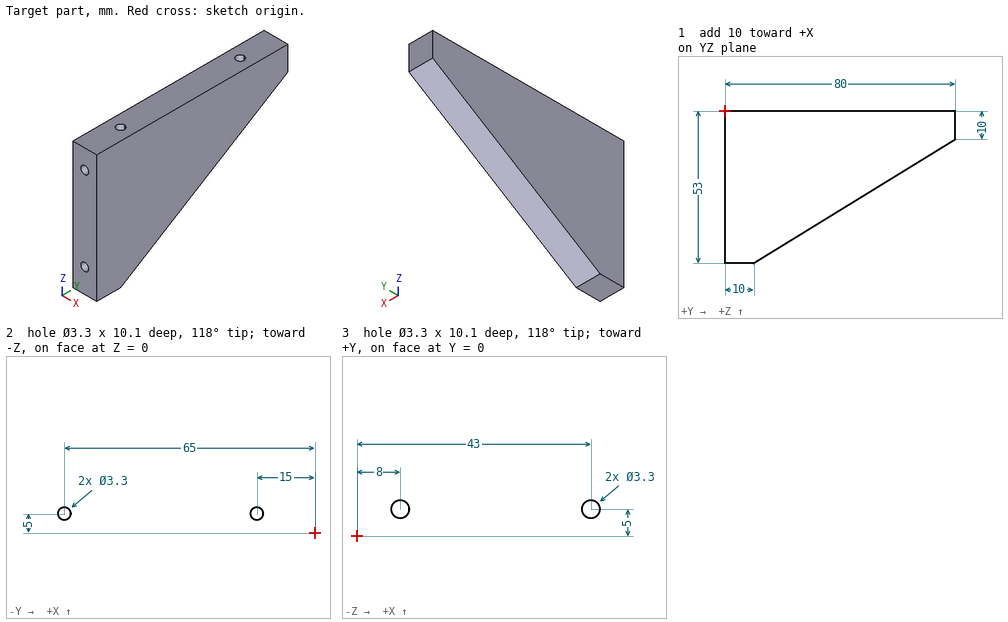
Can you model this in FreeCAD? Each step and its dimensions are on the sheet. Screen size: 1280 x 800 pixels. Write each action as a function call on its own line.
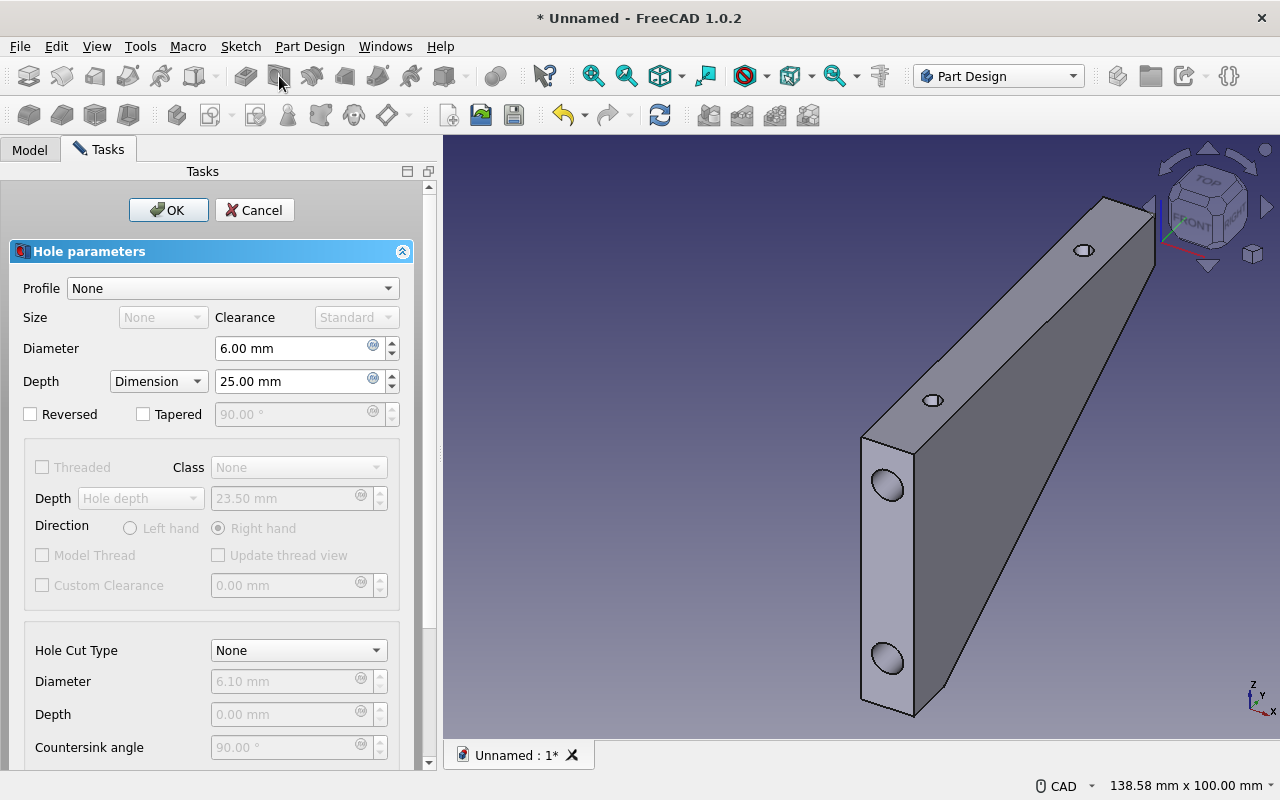
triple_click(300, 348)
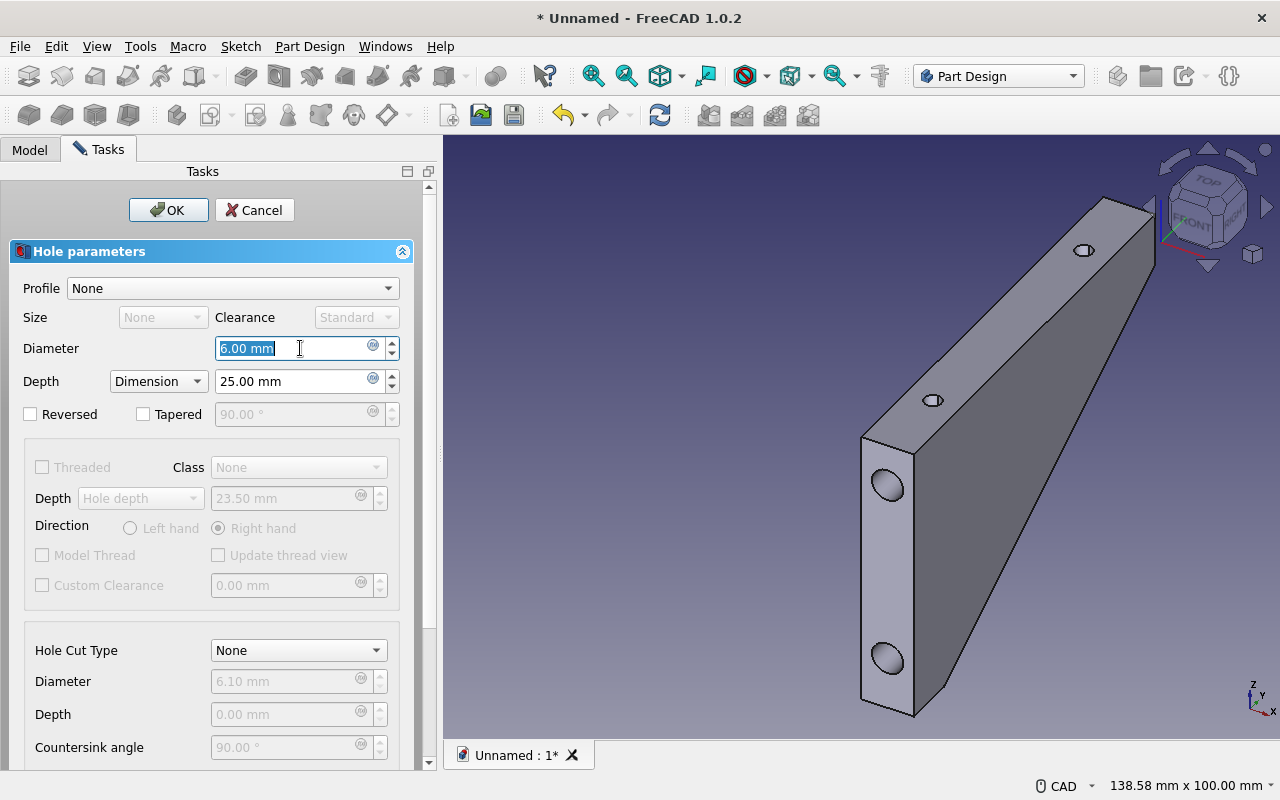
text(3.3)
key(Tab)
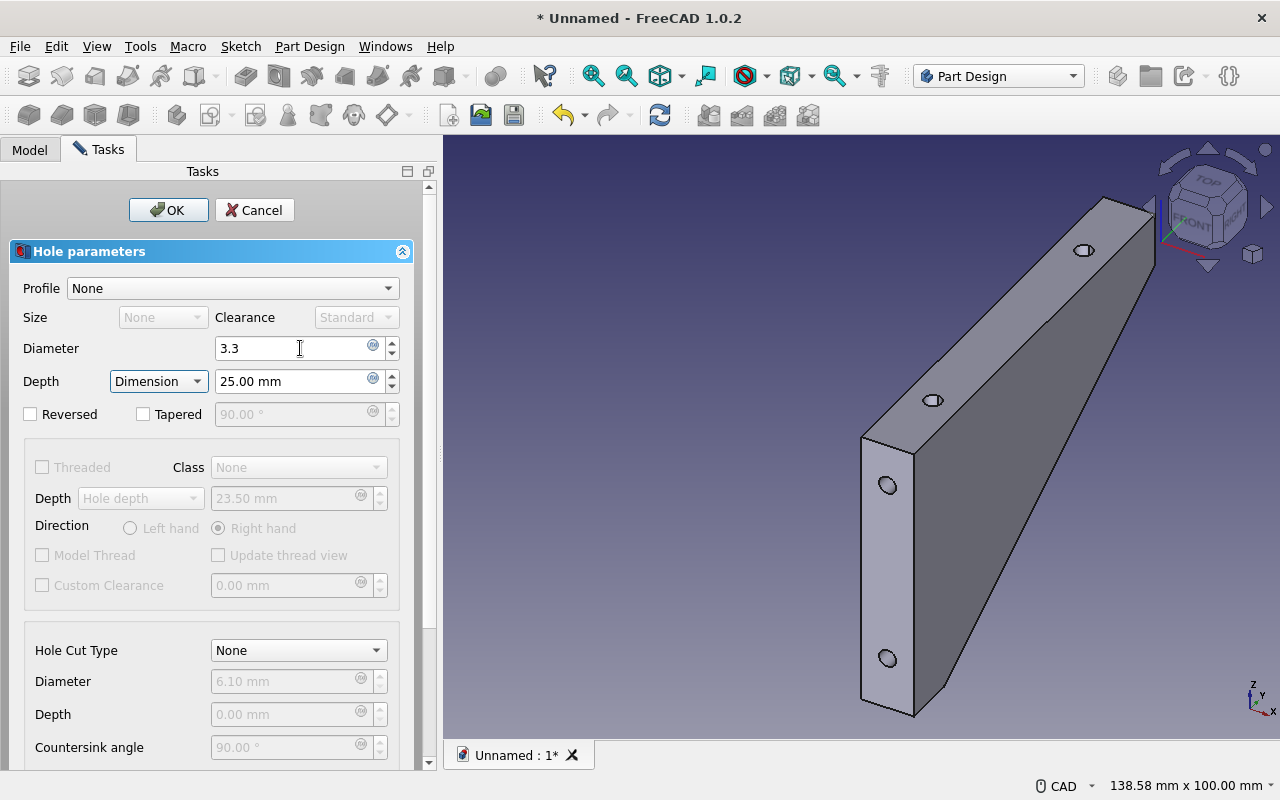
triple_click(300, 382)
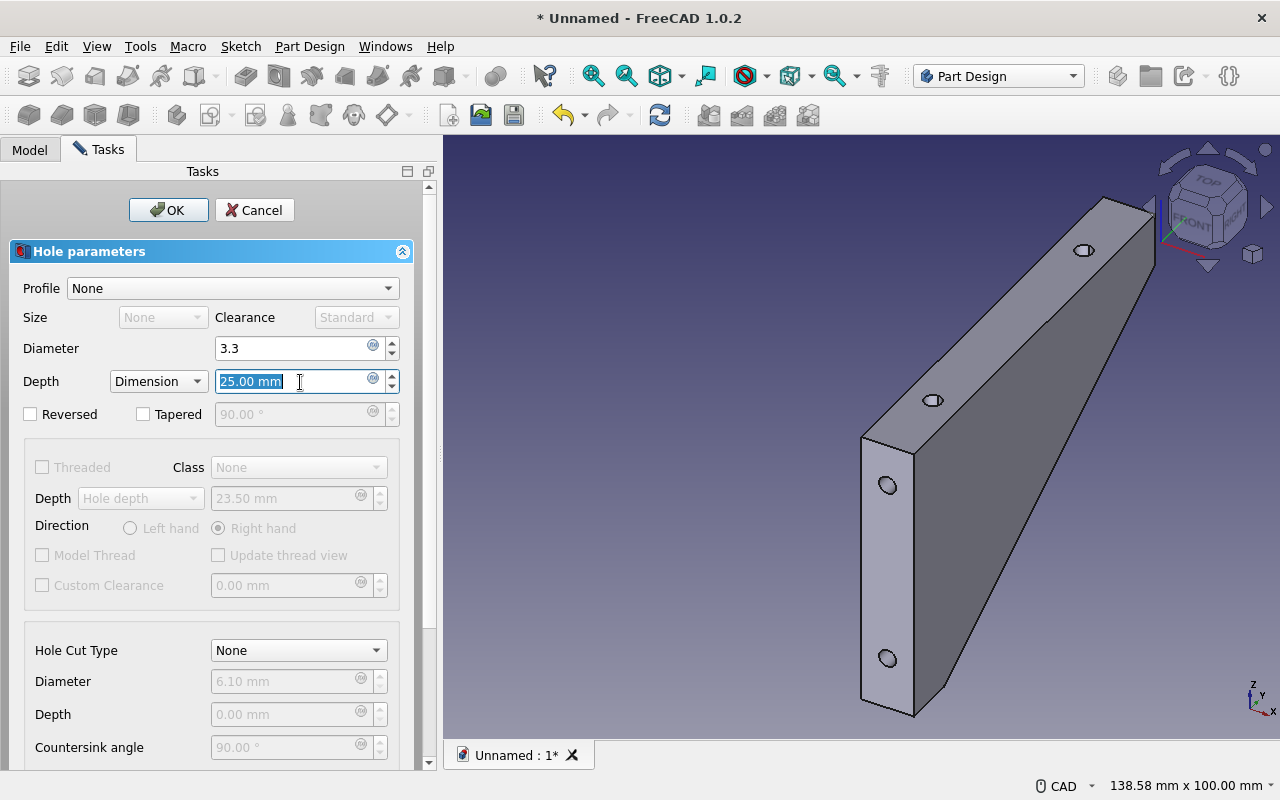
text(10.1)
key(Tab)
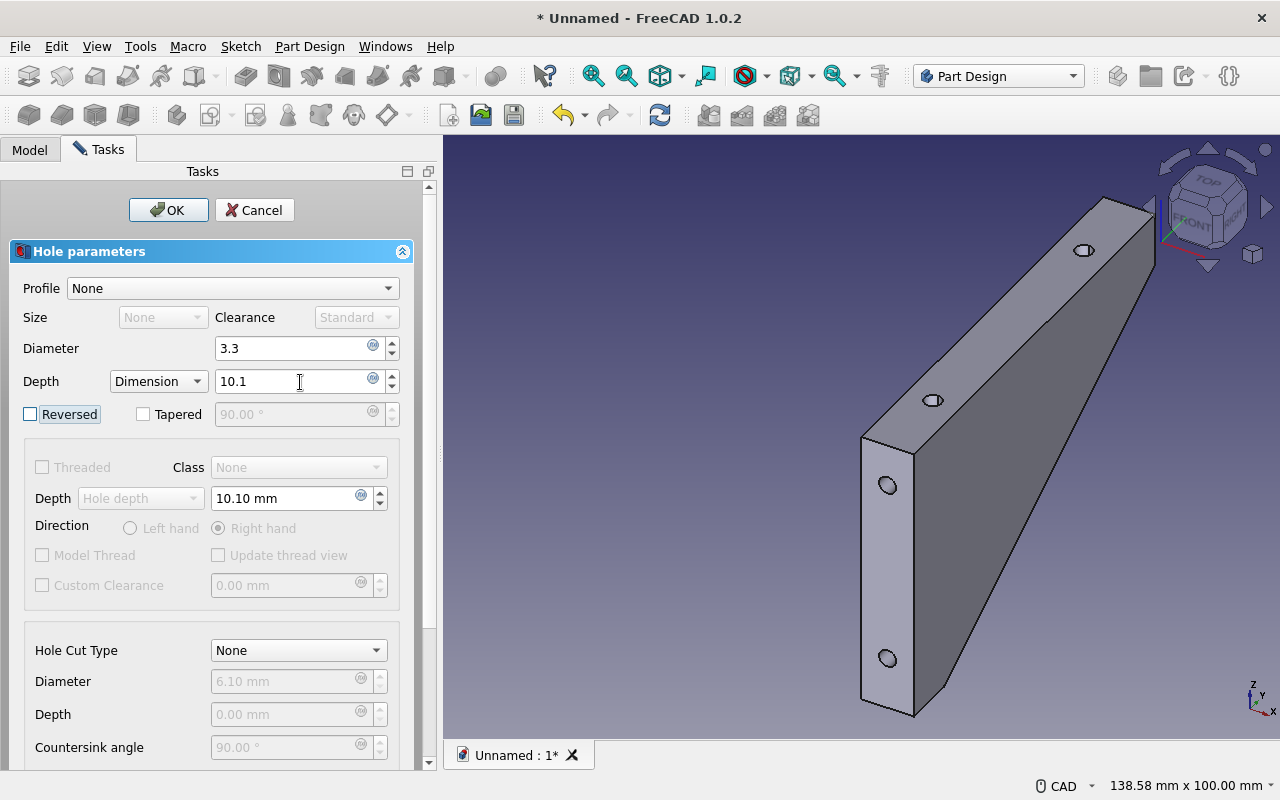
click(169, 210)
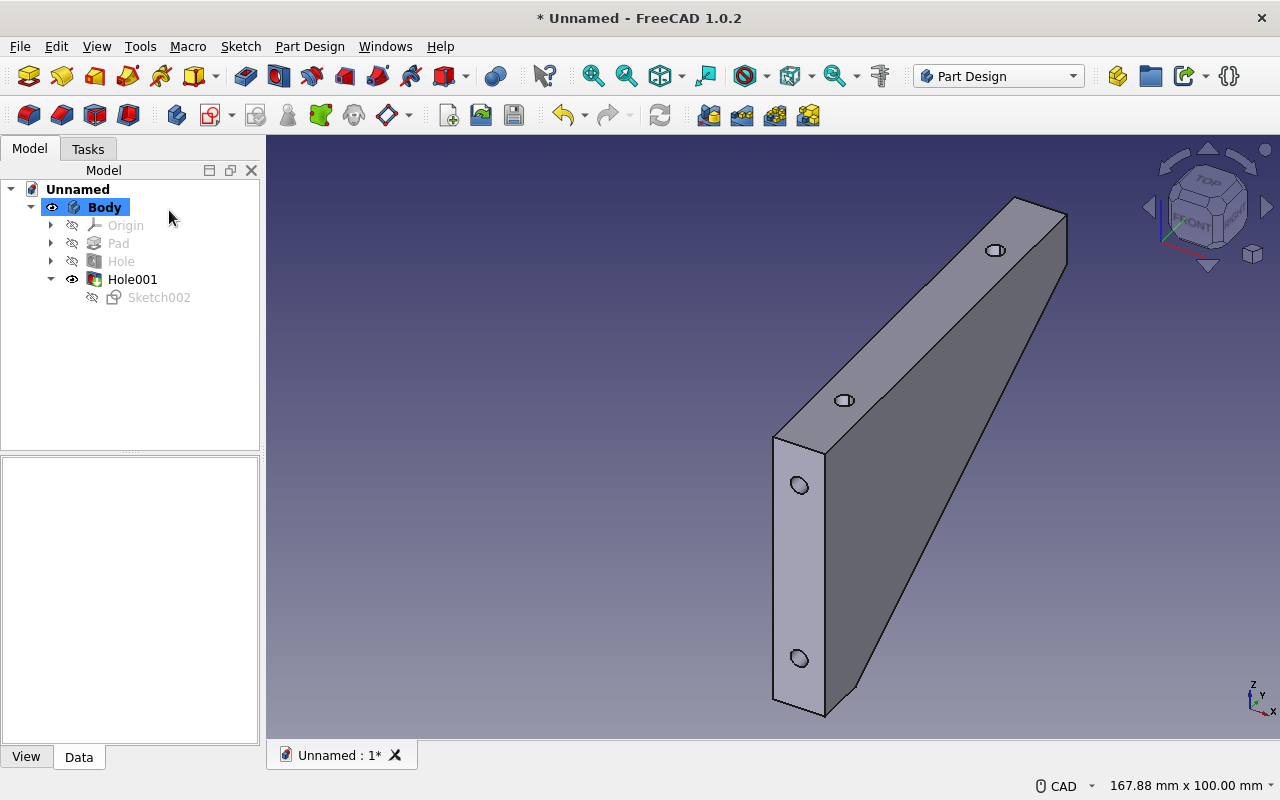
key(0)